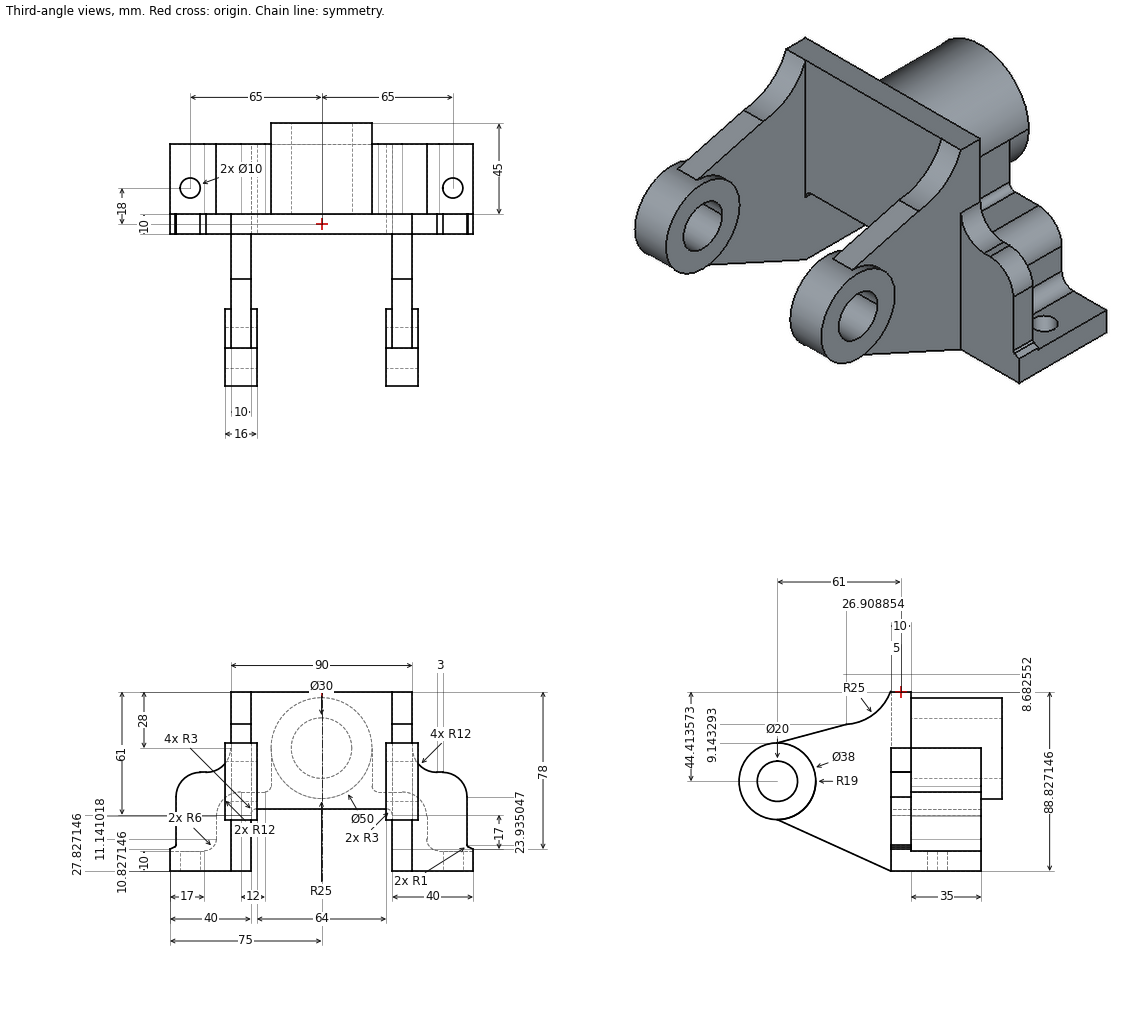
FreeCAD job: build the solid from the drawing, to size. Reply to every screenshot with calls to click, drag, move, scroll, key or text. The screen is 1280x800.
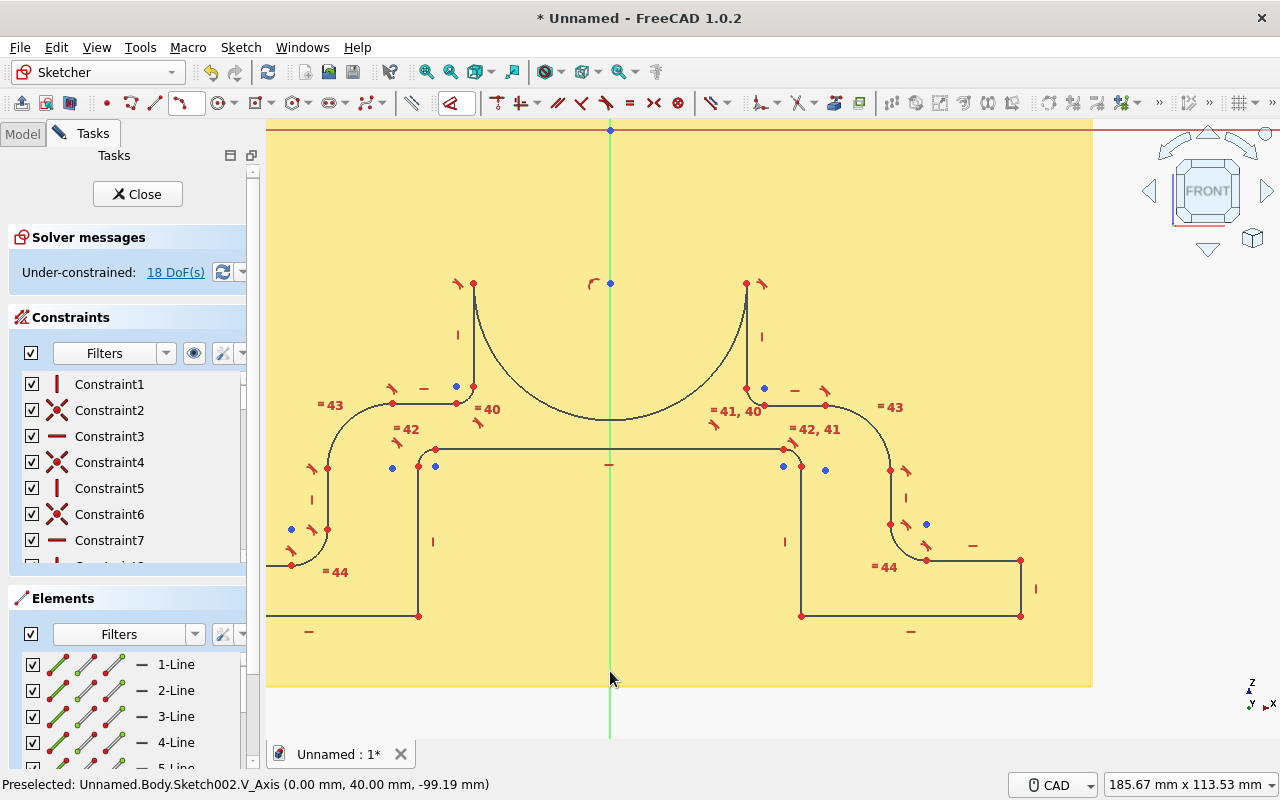
click(393, 469)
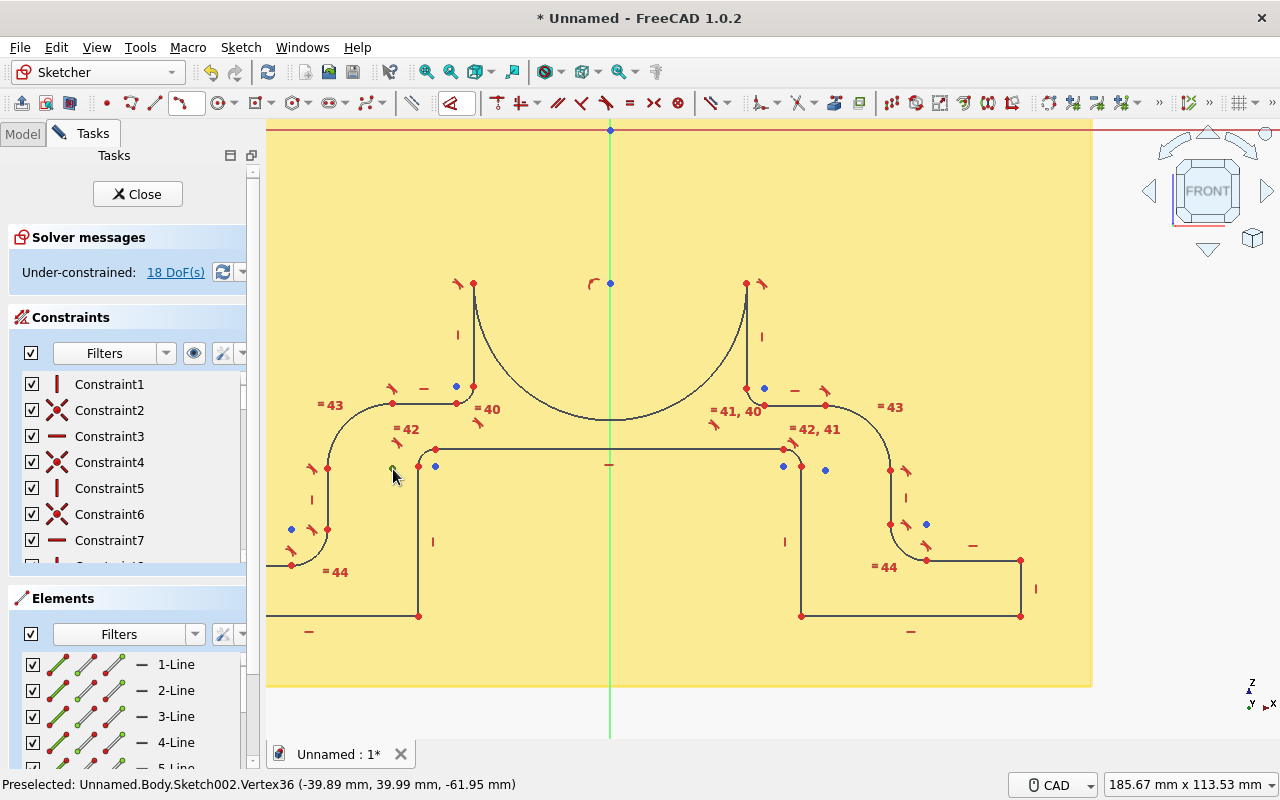
click(826, 471)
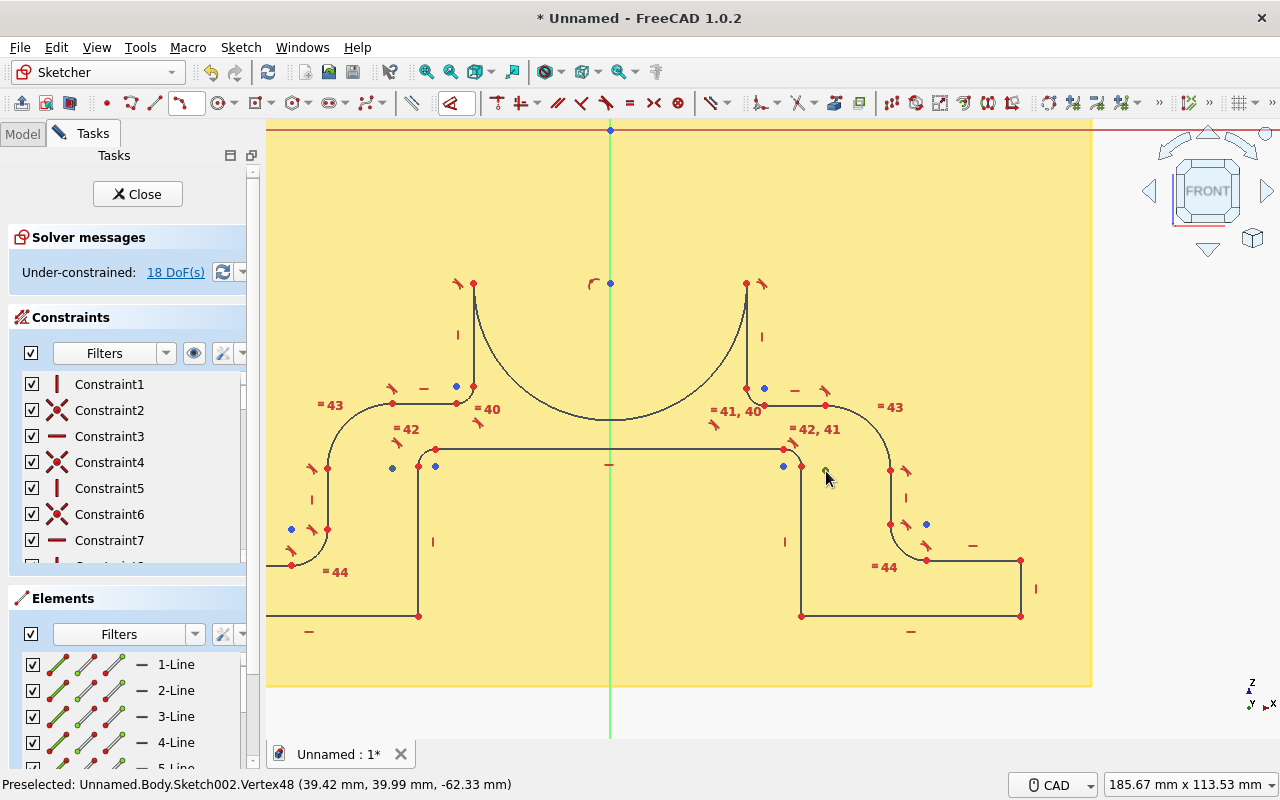
click(610, 671)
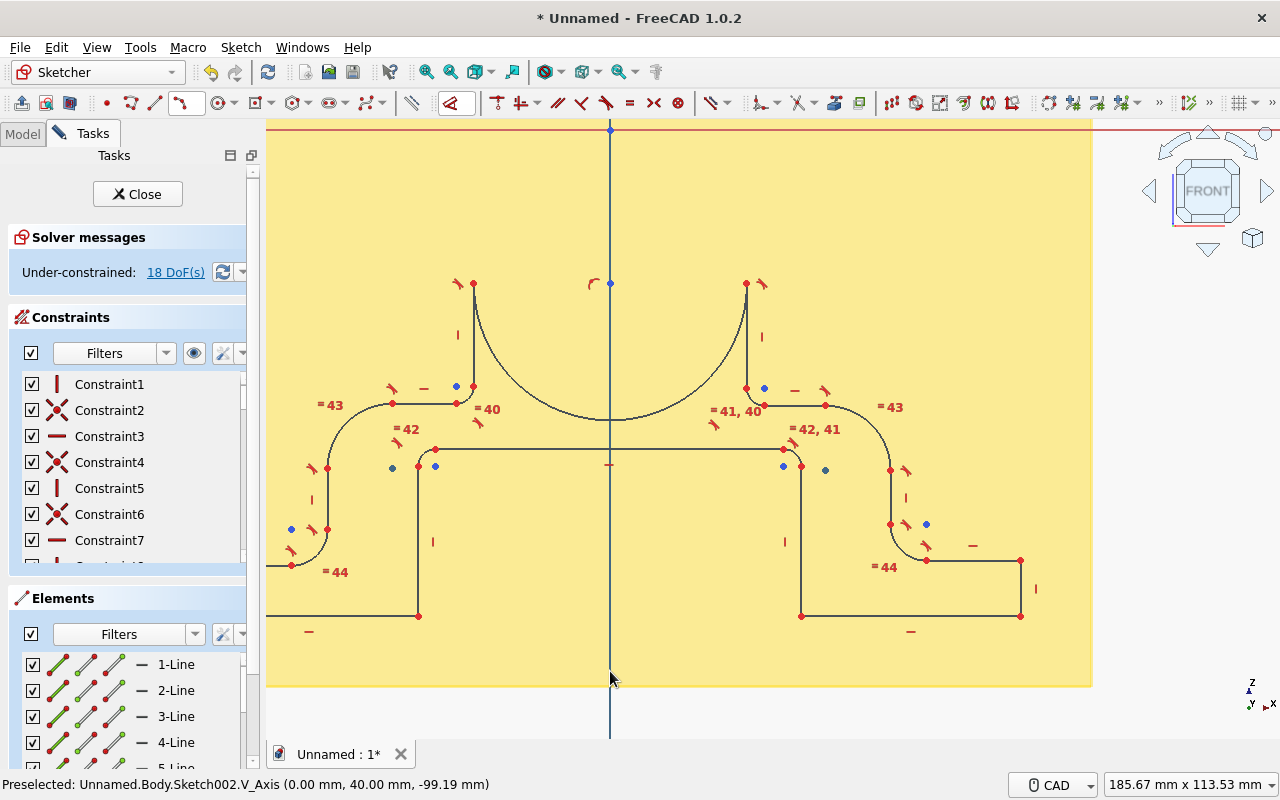
key(s)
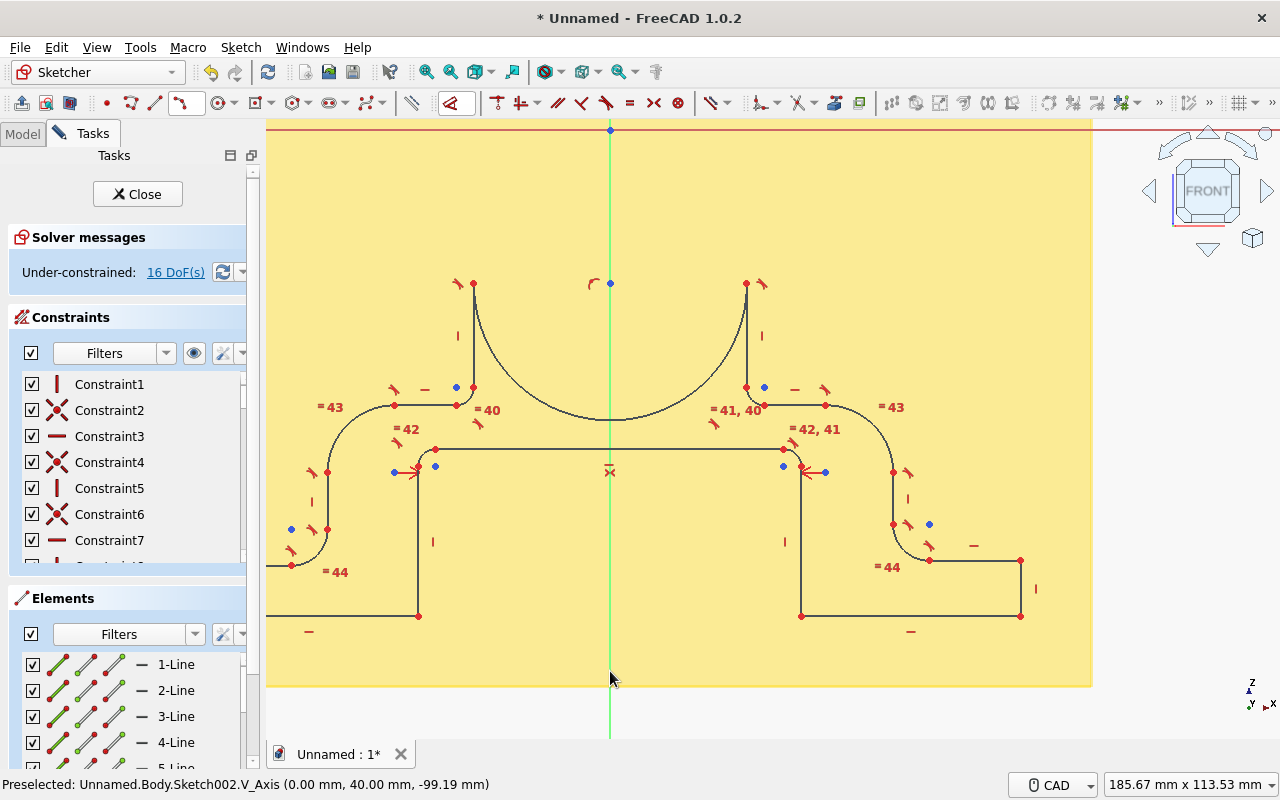
scroll(896, 543, down, 2)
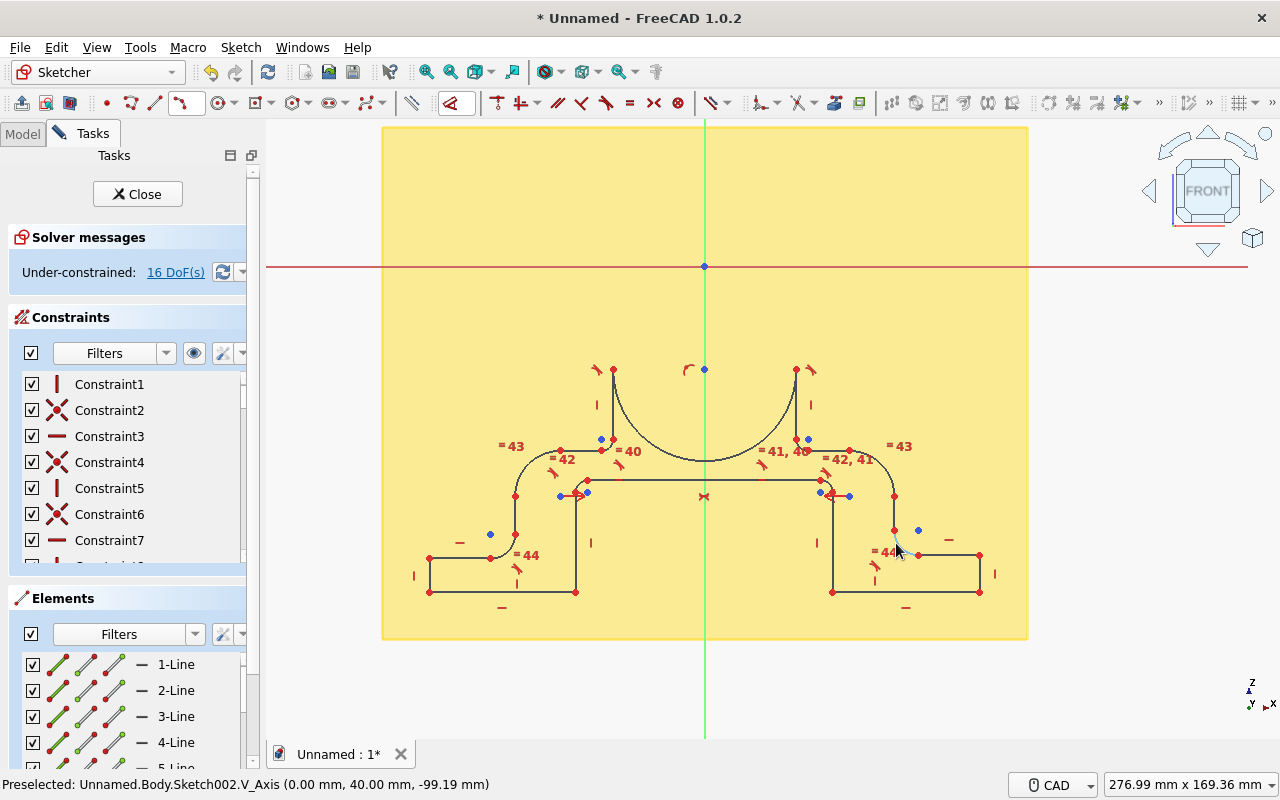
click(430, 558)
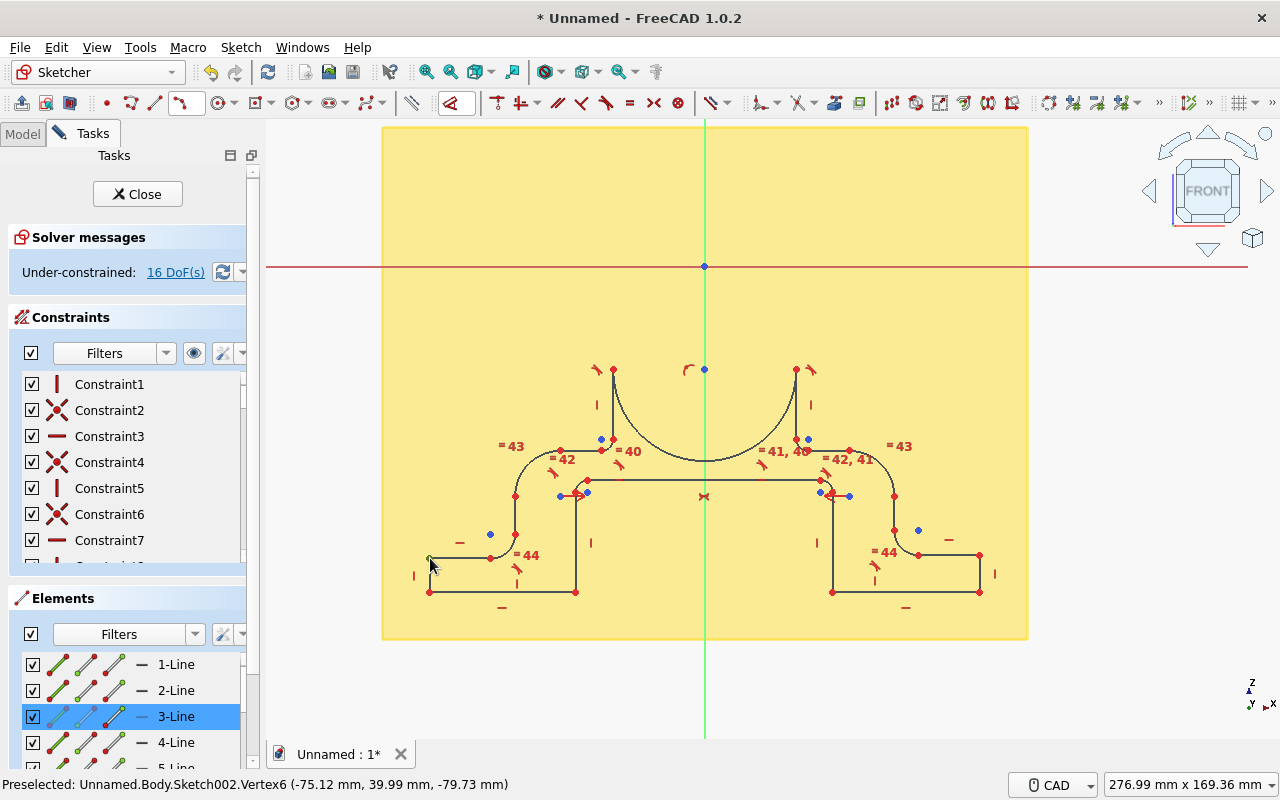
click(980, 555)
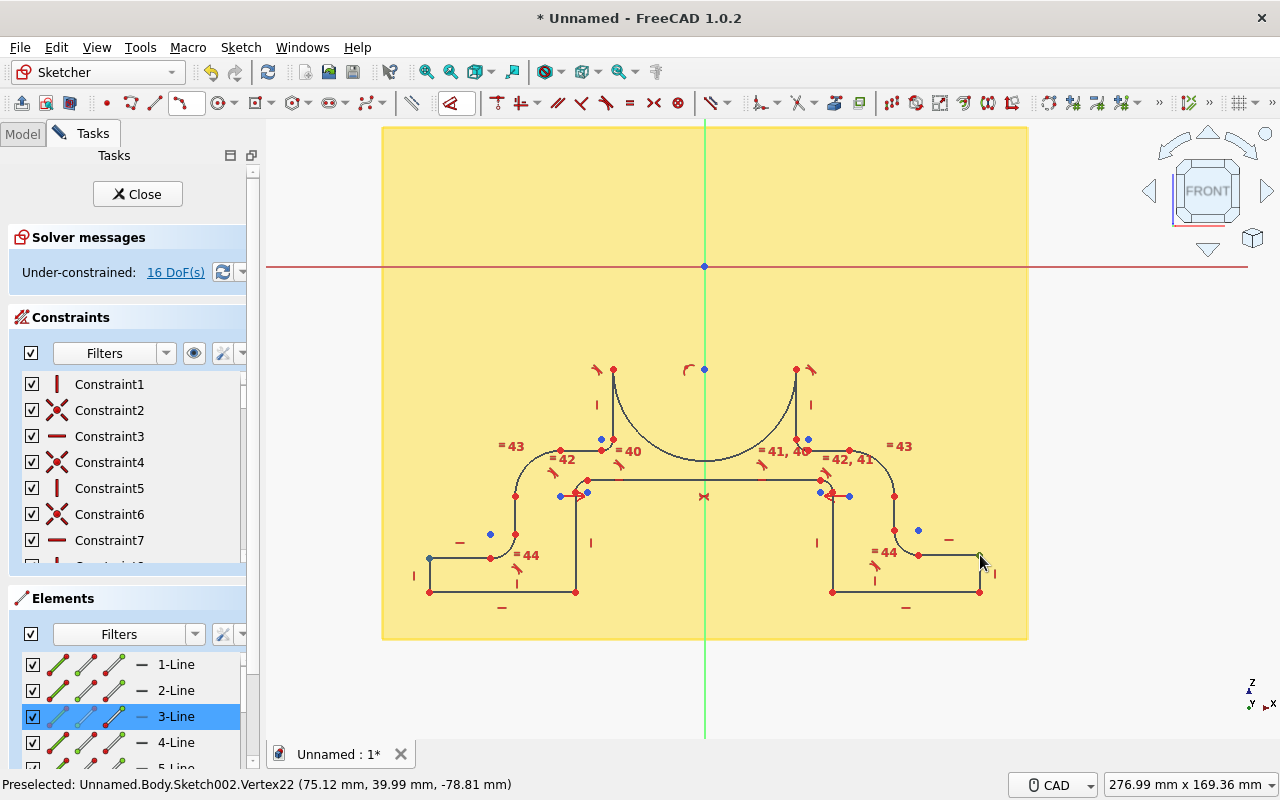
click(705, 671)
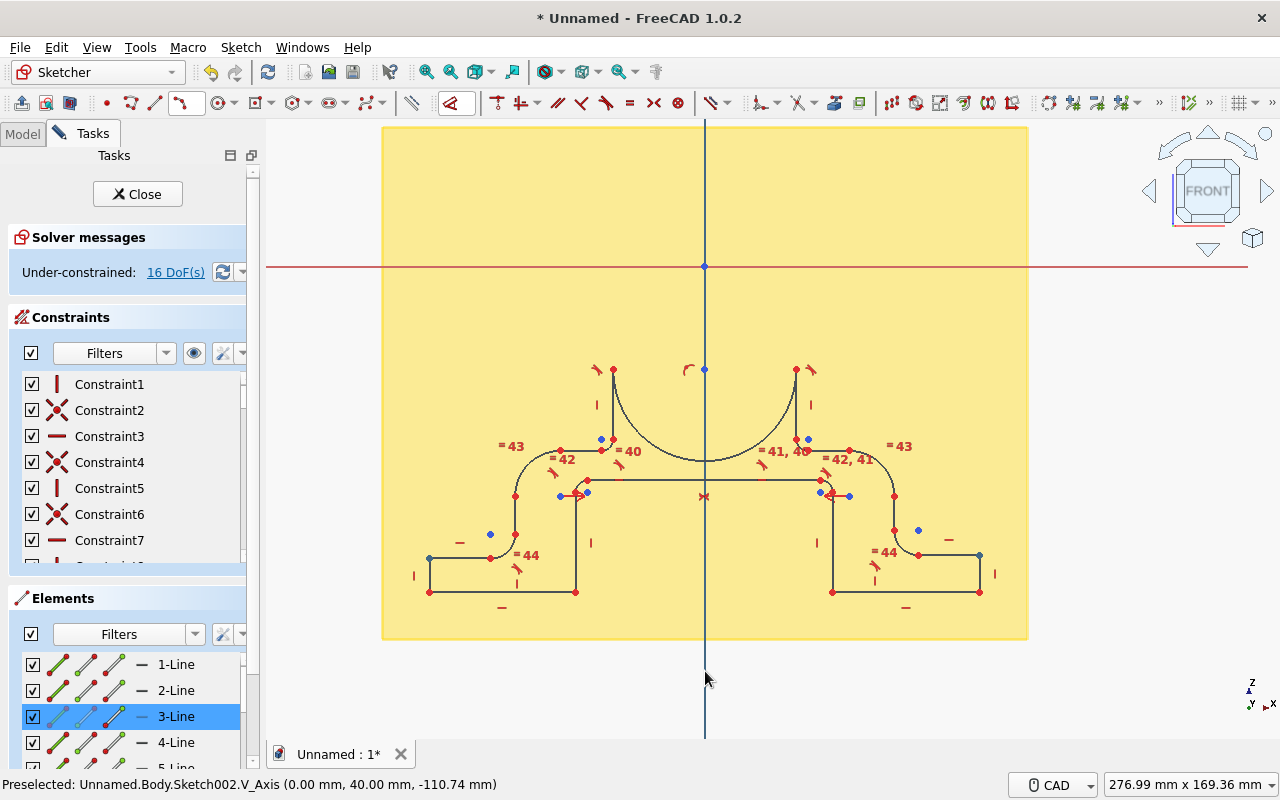
click(654, 104)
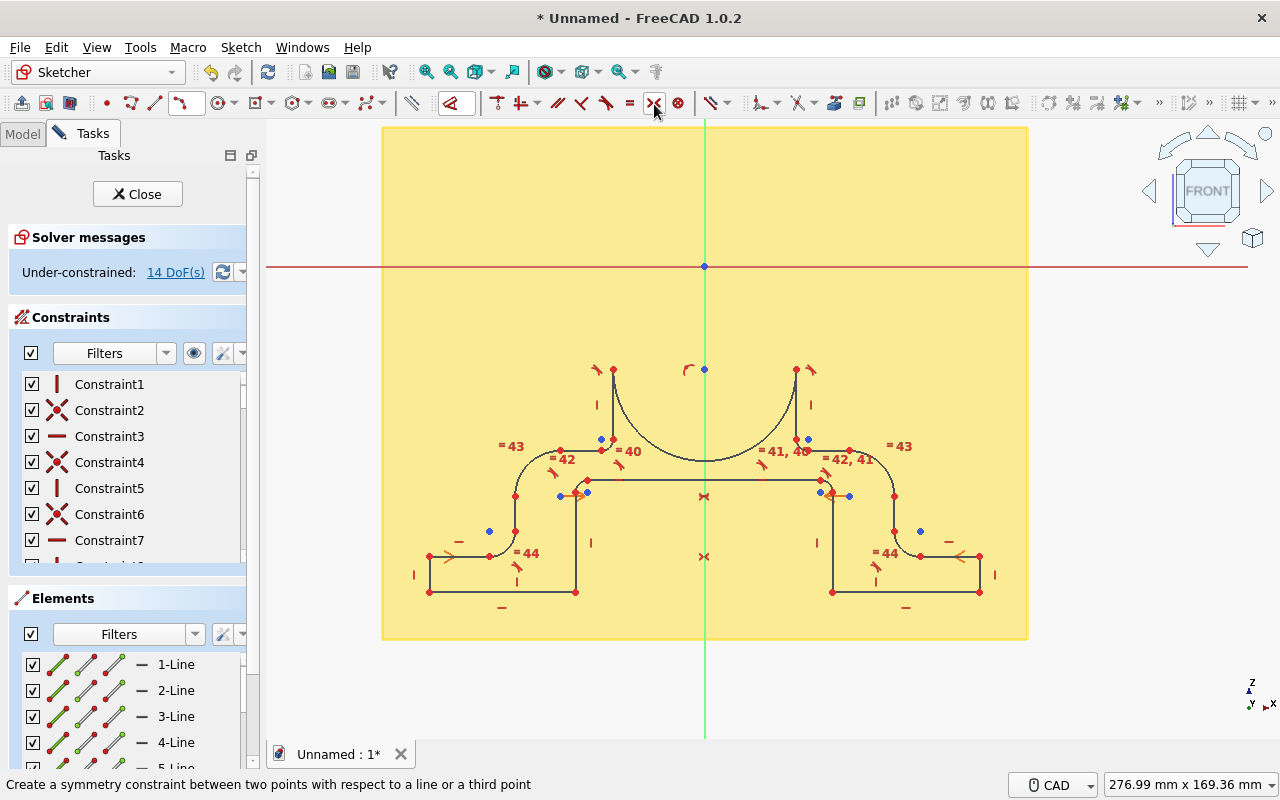
click(576, 592)